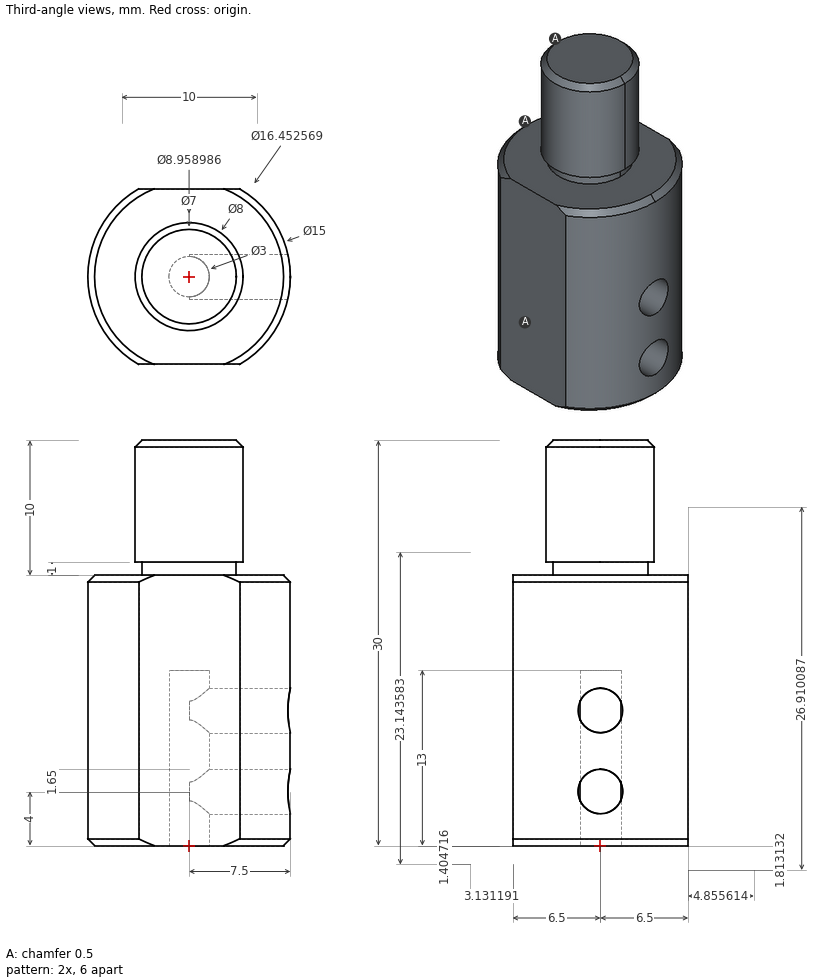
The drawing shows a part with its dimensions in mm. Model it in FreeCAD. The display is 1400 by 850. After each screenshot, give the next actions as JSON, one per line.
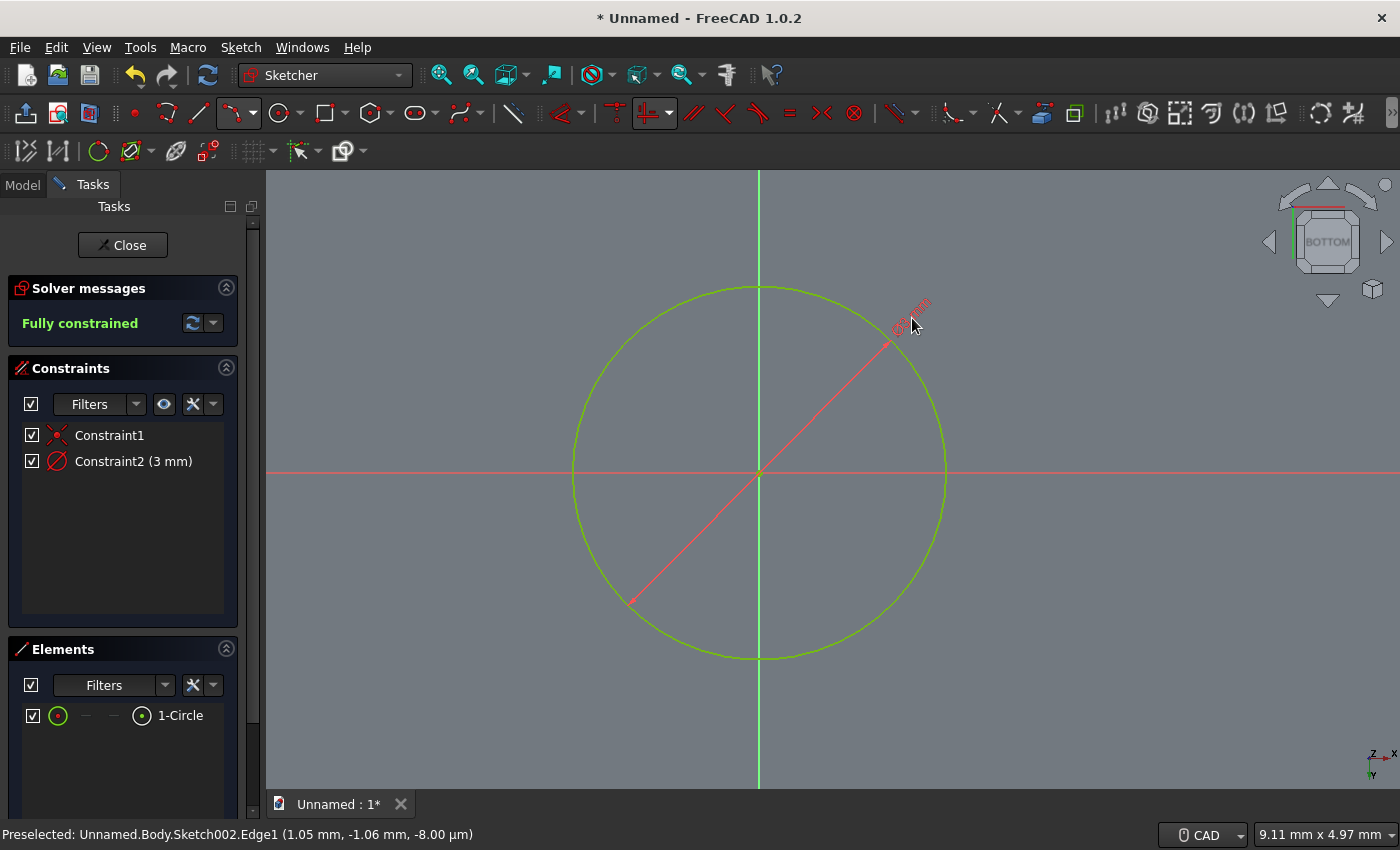
{"action": "left_click", "coordinate": [123, 245]}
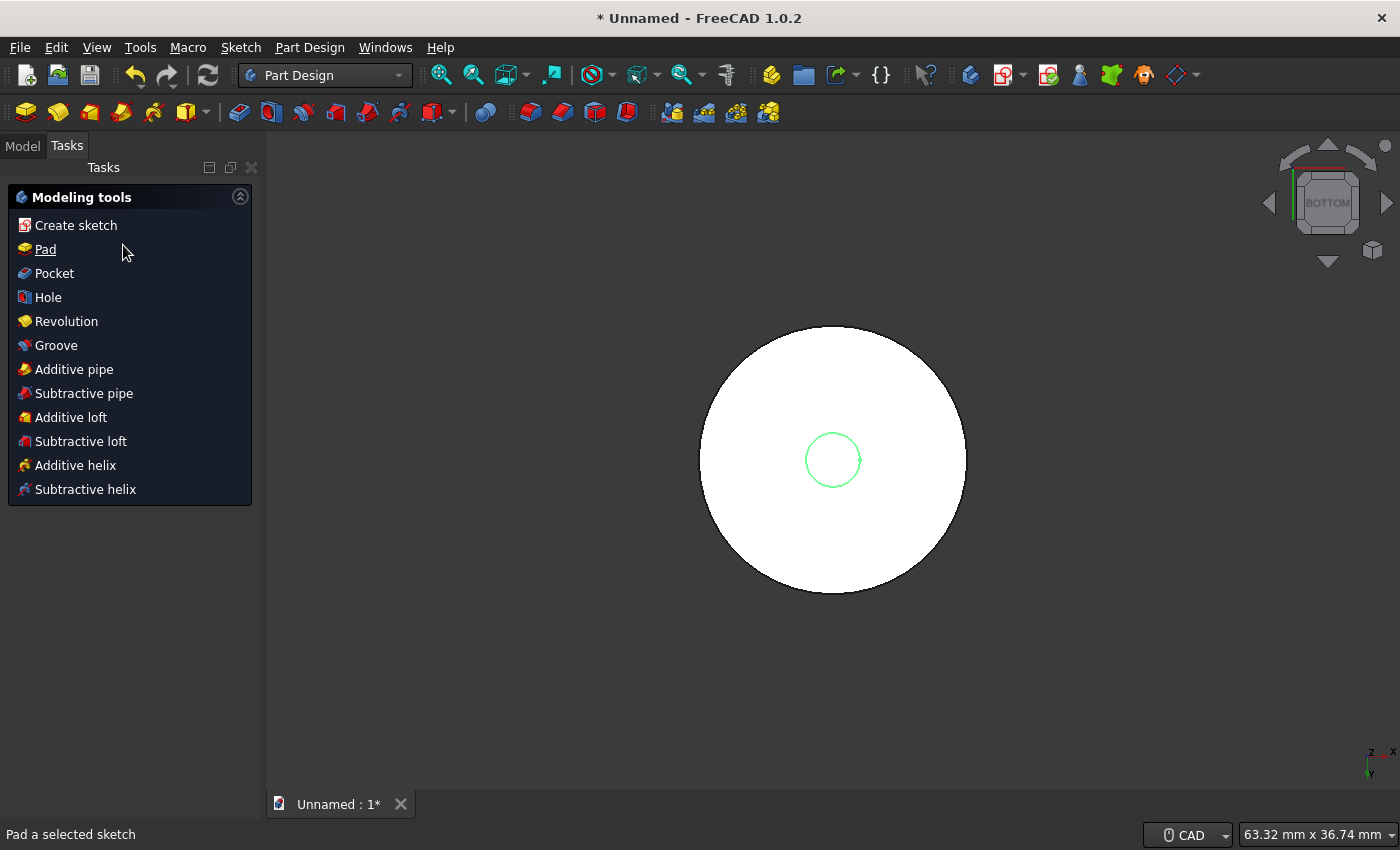
{"action": "left_click", "coordinate": [240, 112]}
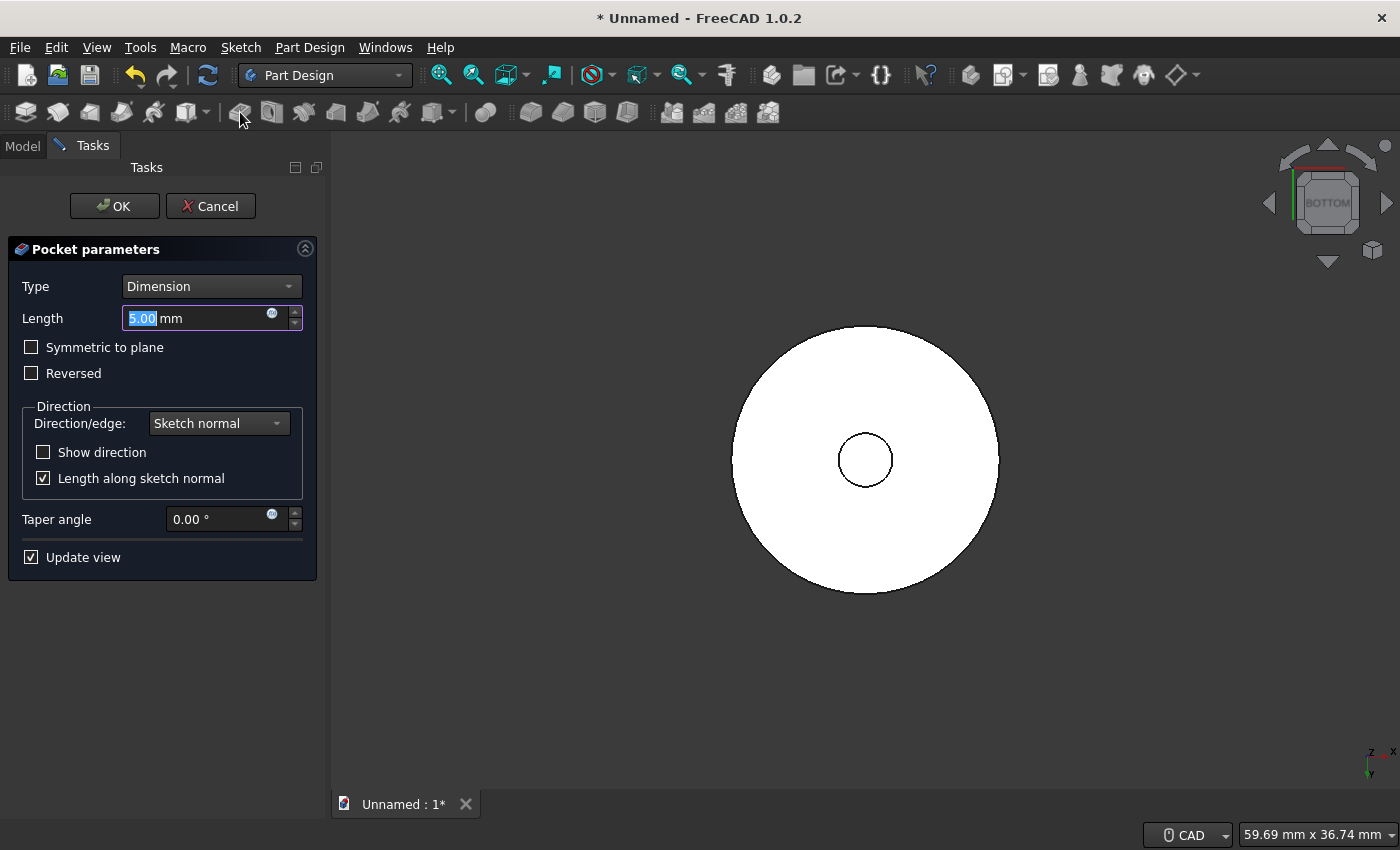
{"action": "type", "text": "13"}
{"action": "key", "text": "Tab"}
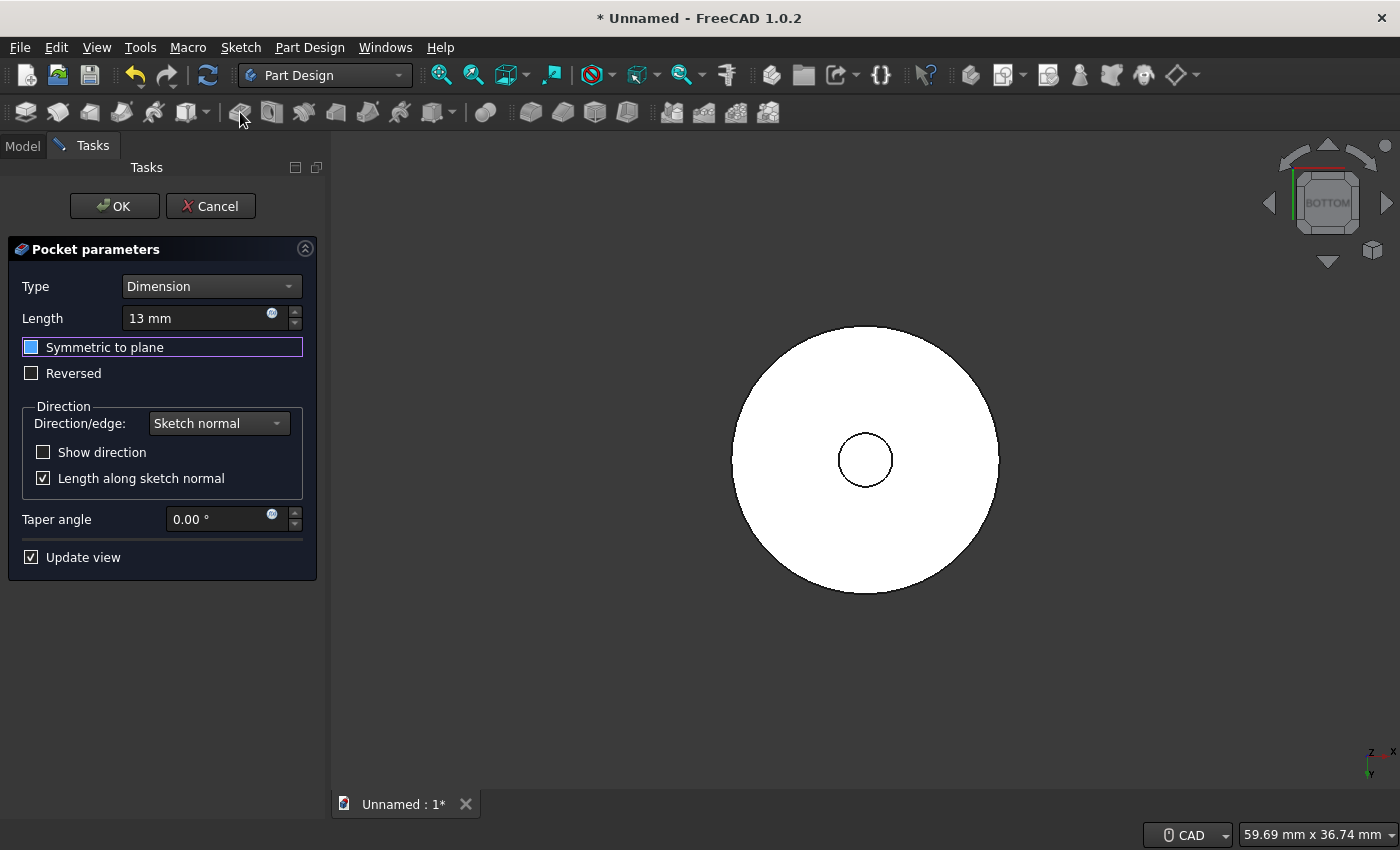
{"action": "left_click", "coordinate": [115, 206]}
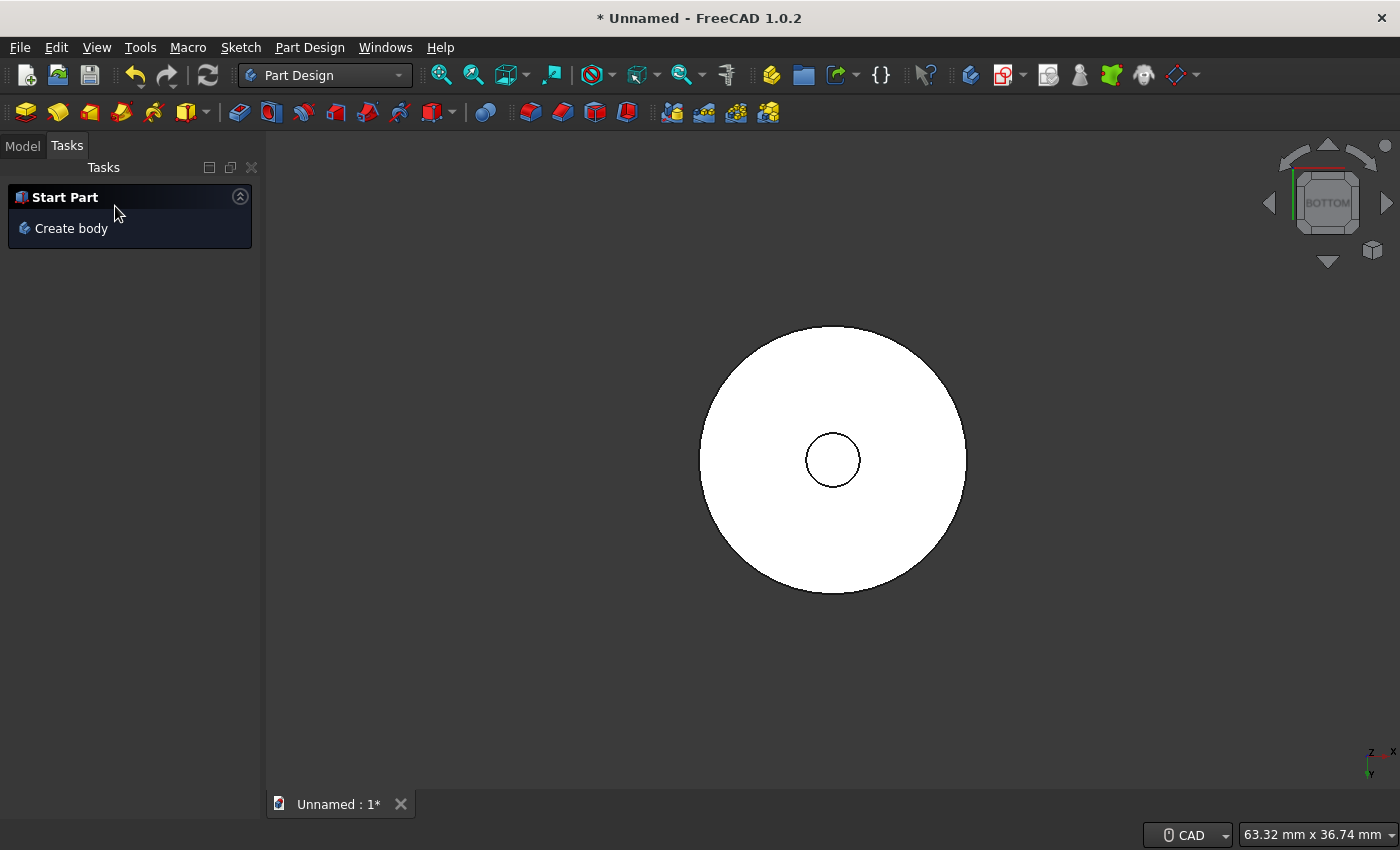
{"action": "left_click", "coordinate": [442, 76]}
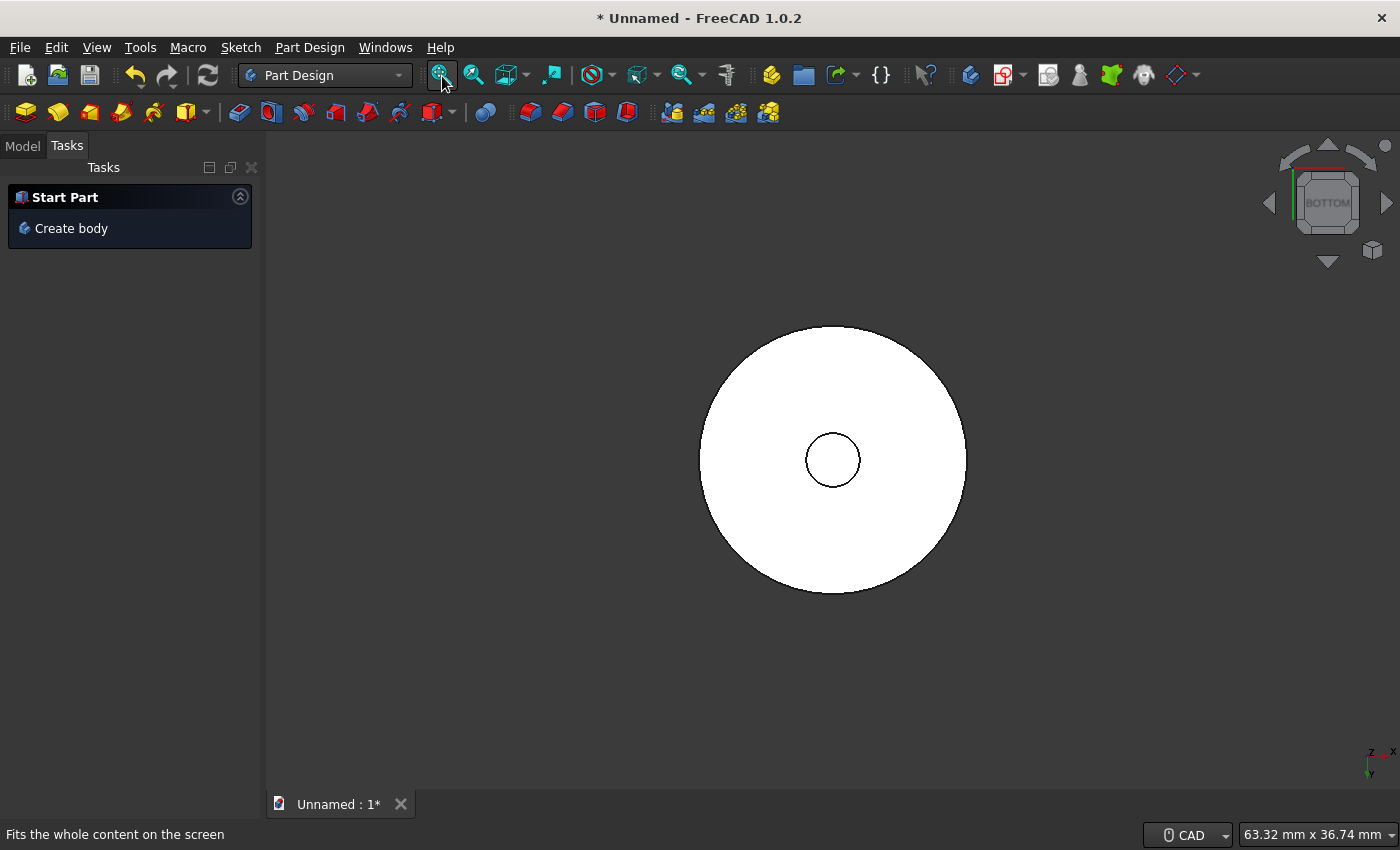
{"action": "key", "text": "0"}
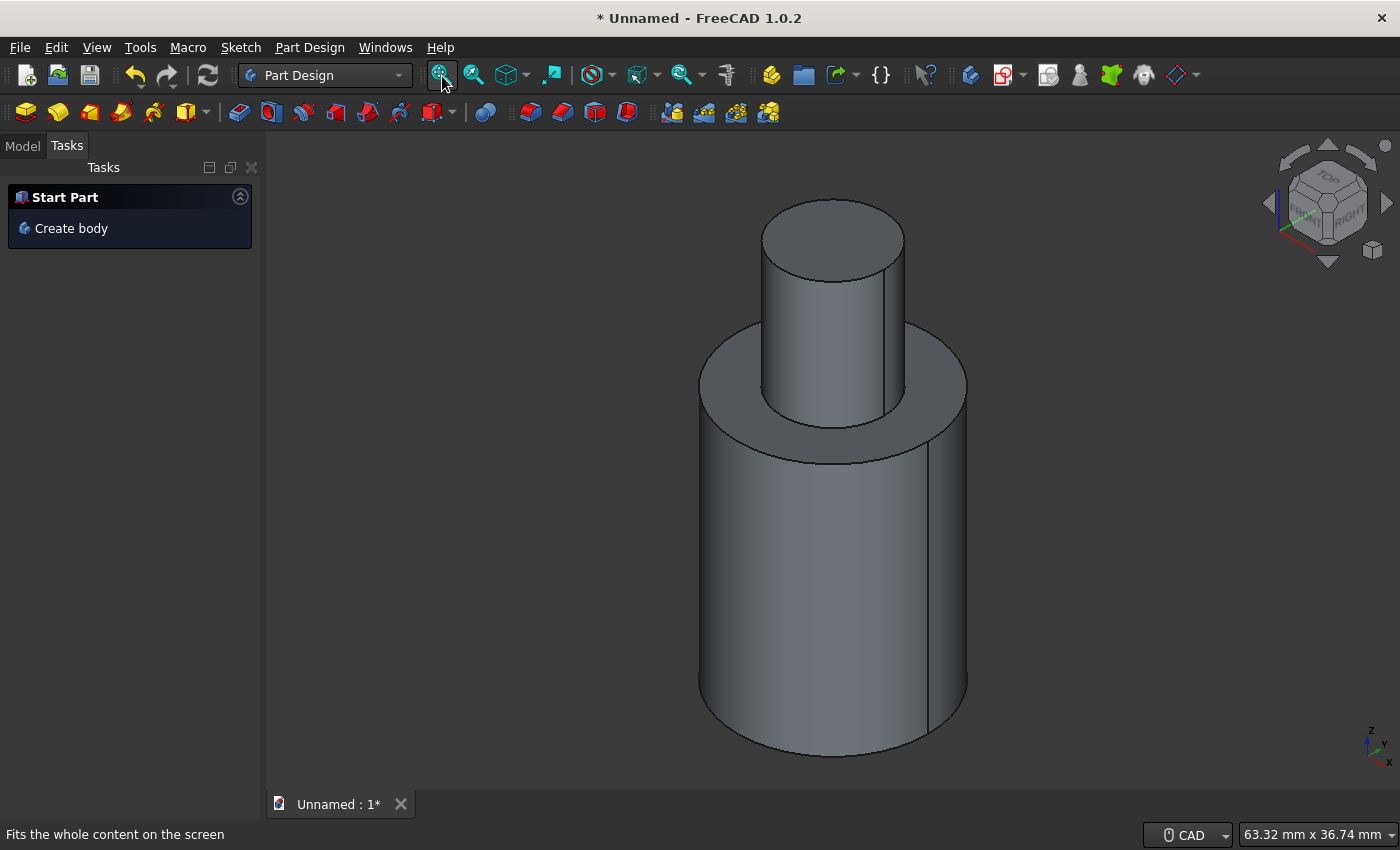
{"action": "left_click", "coordinate": [442, 76]}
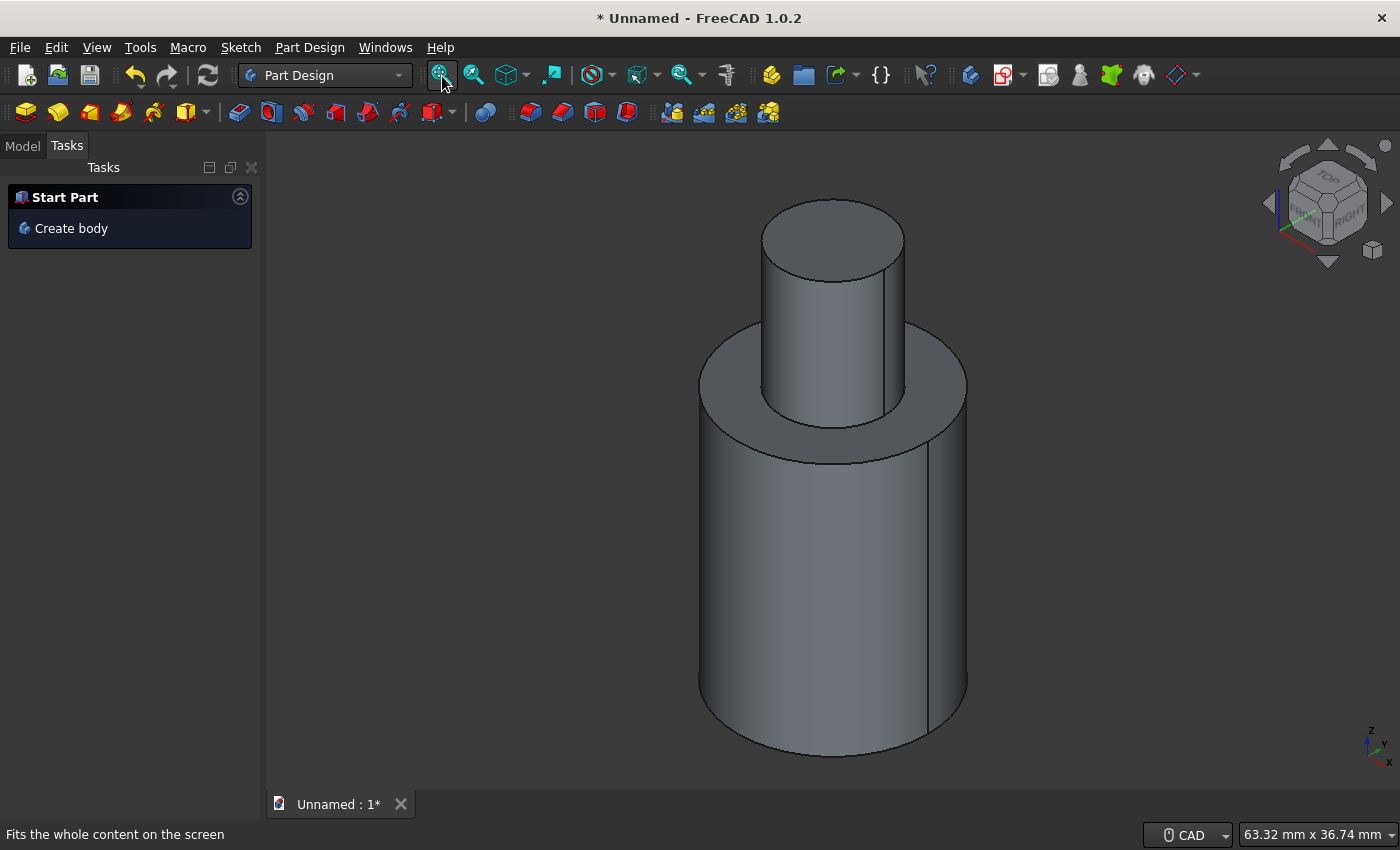
{"action": "left_click", "coordinate": [724, 386]}